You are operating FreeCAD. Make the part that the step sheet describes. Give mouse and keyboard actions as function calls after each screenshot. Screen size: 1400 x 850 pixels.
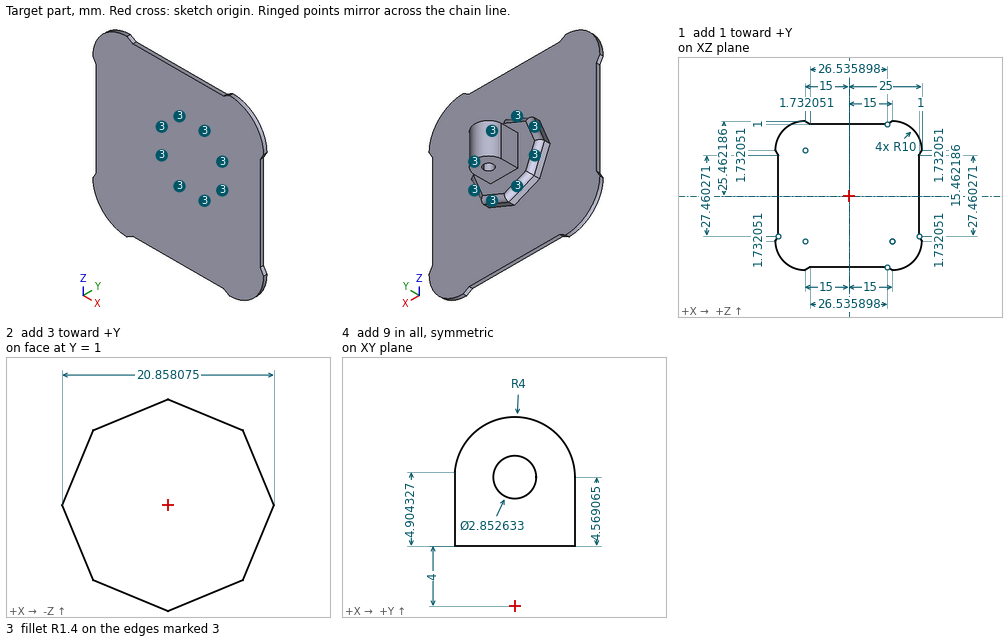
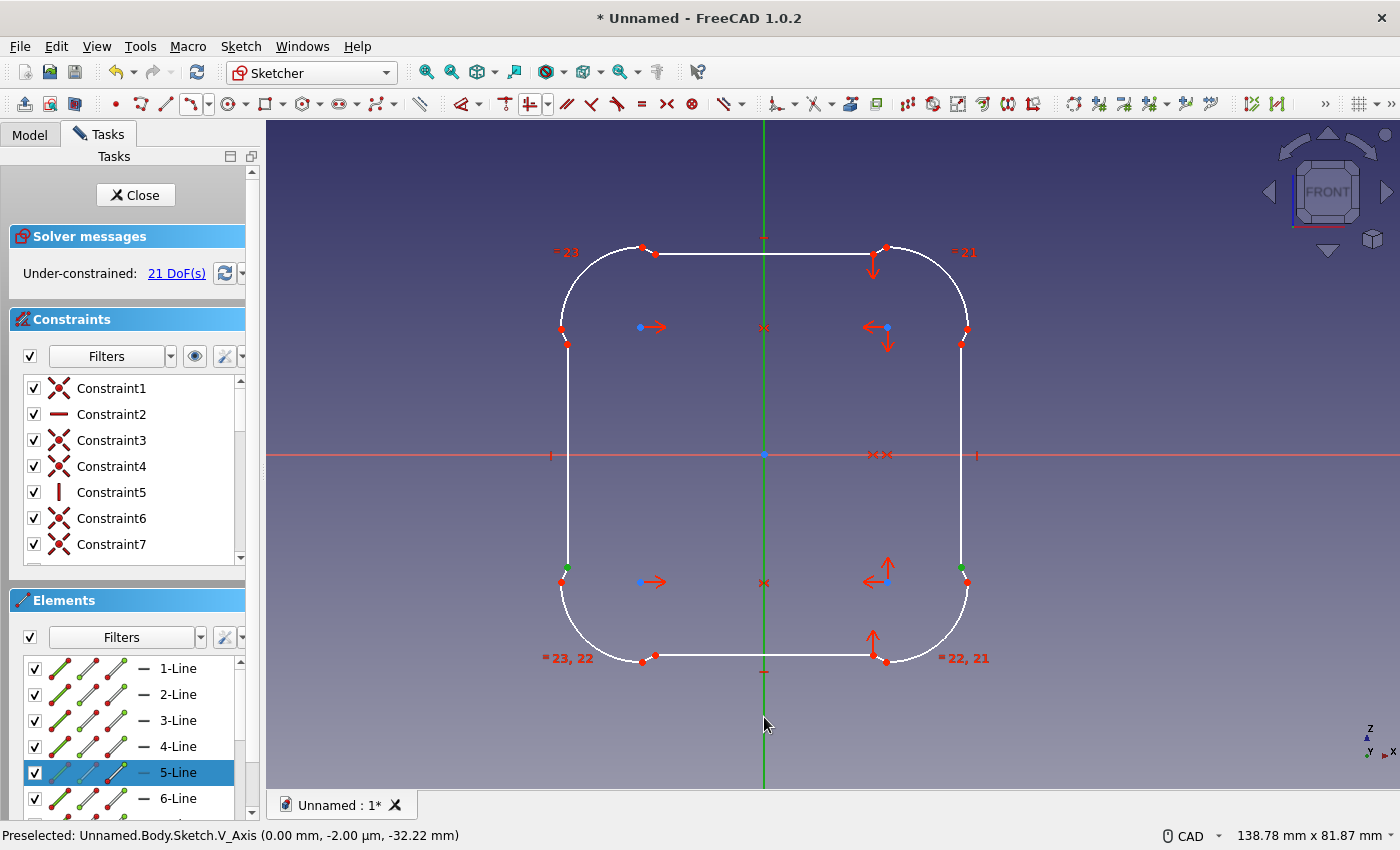
click(667, 104)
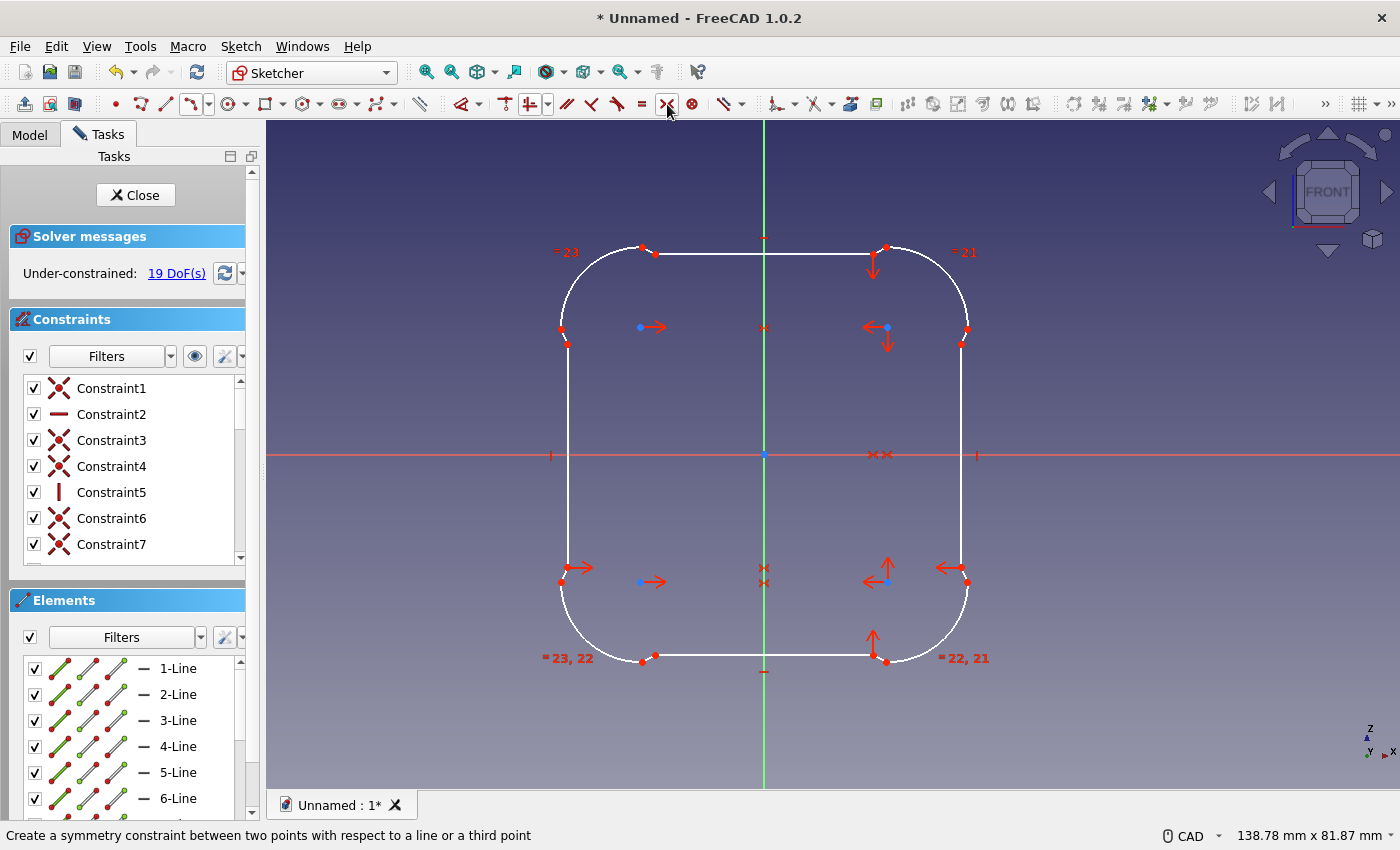
click(460, 104)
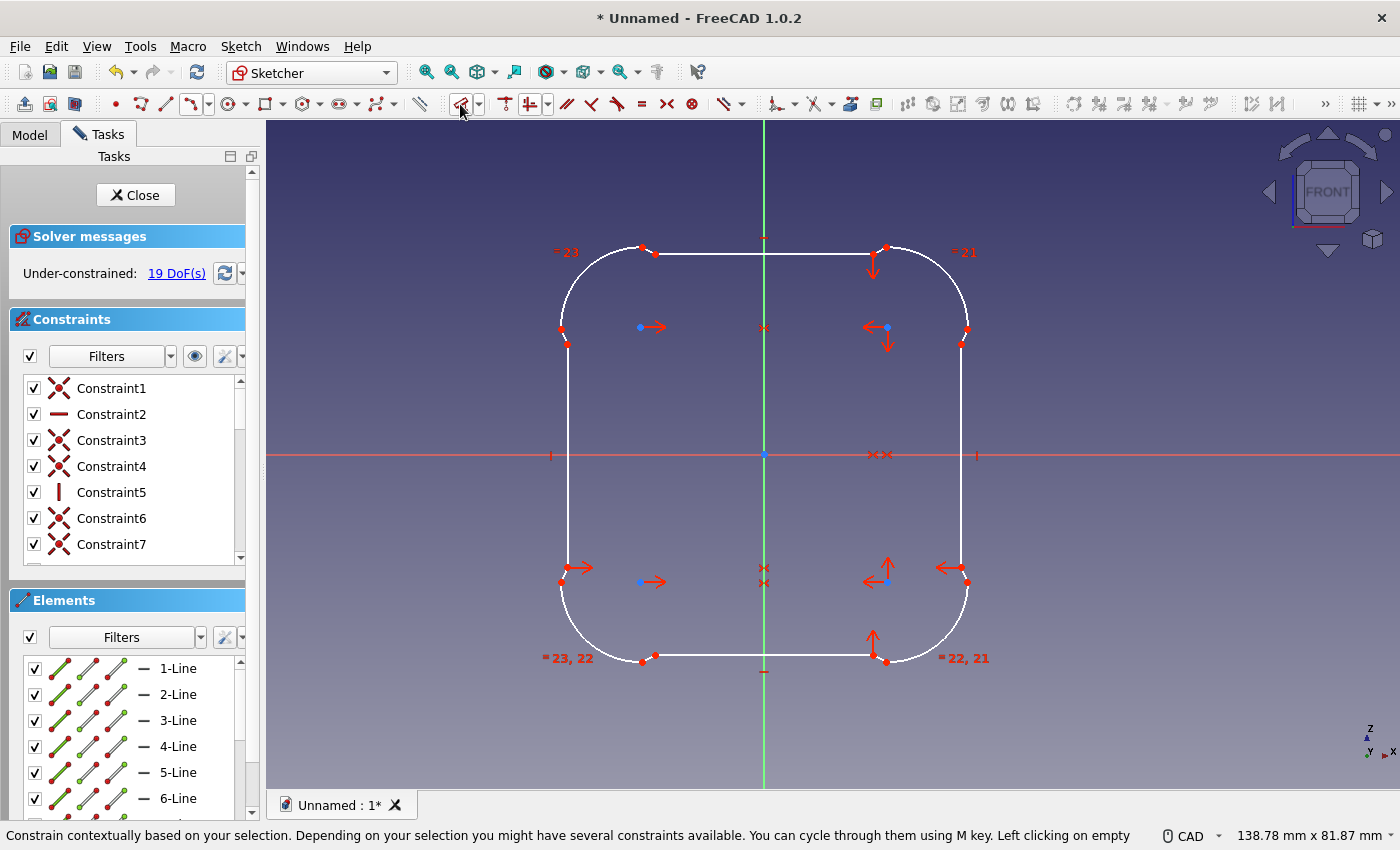
click(960, 292)
click(989, 278)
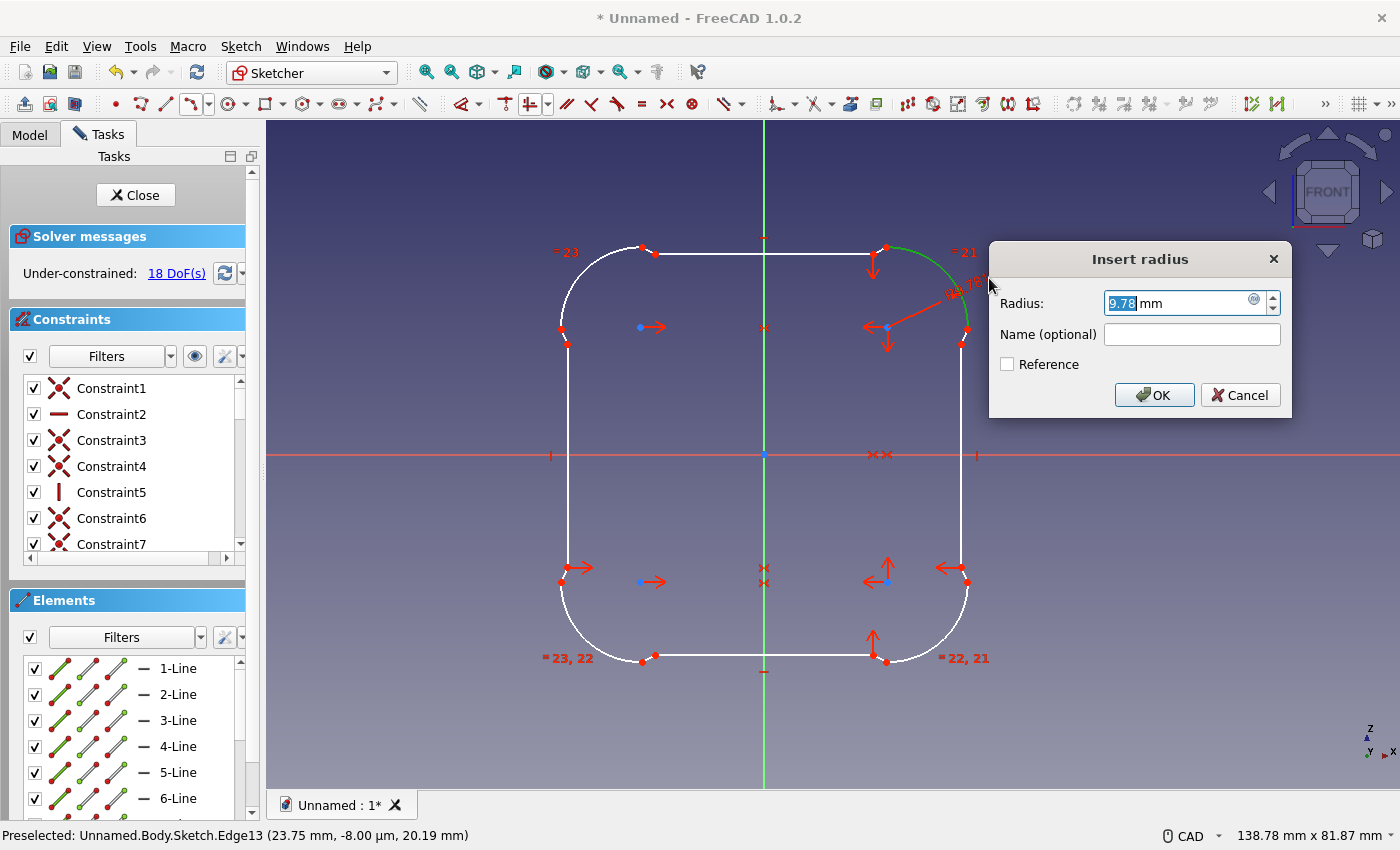
text(10)
key(Return)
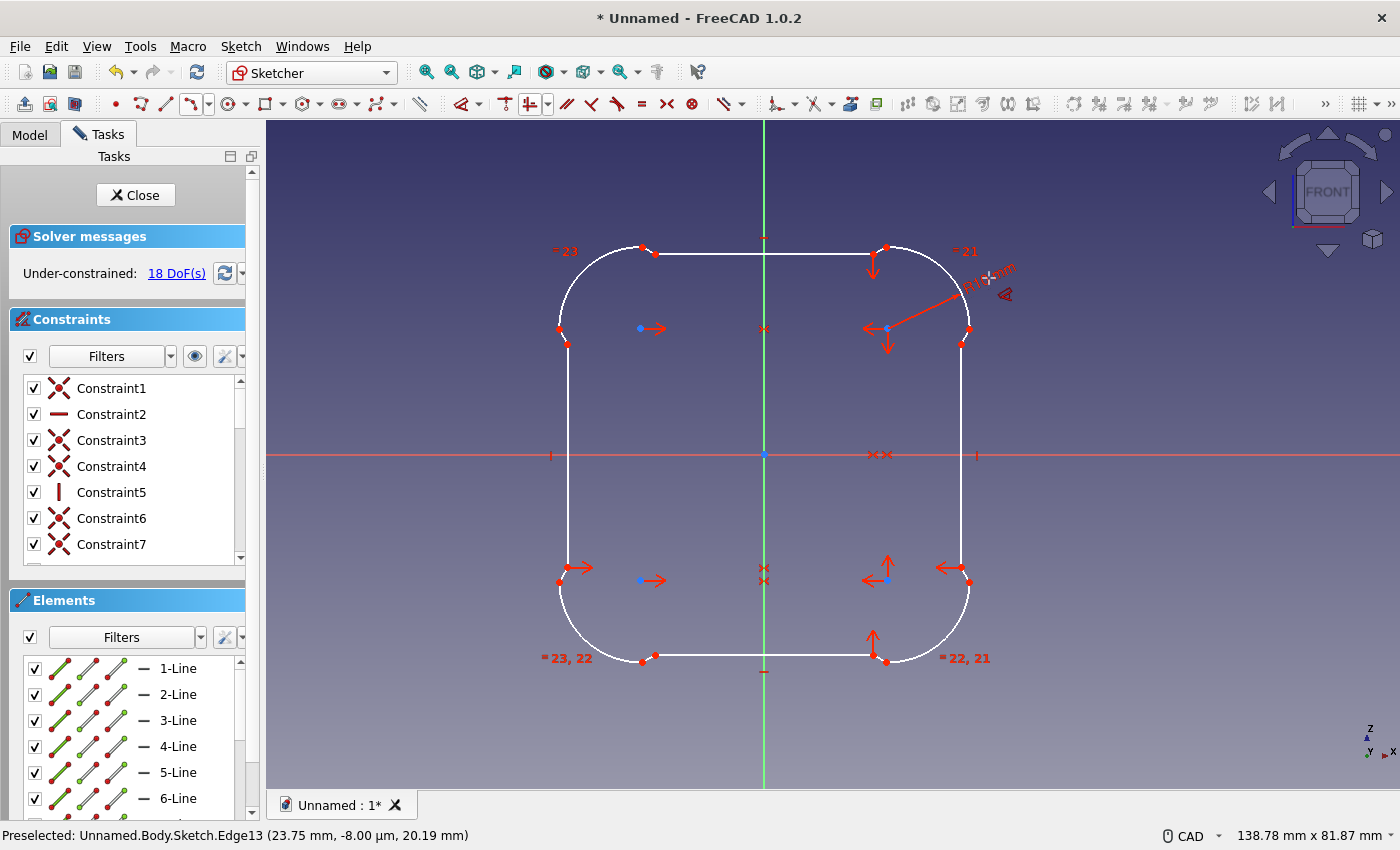
scroll(649, 251, up, 8)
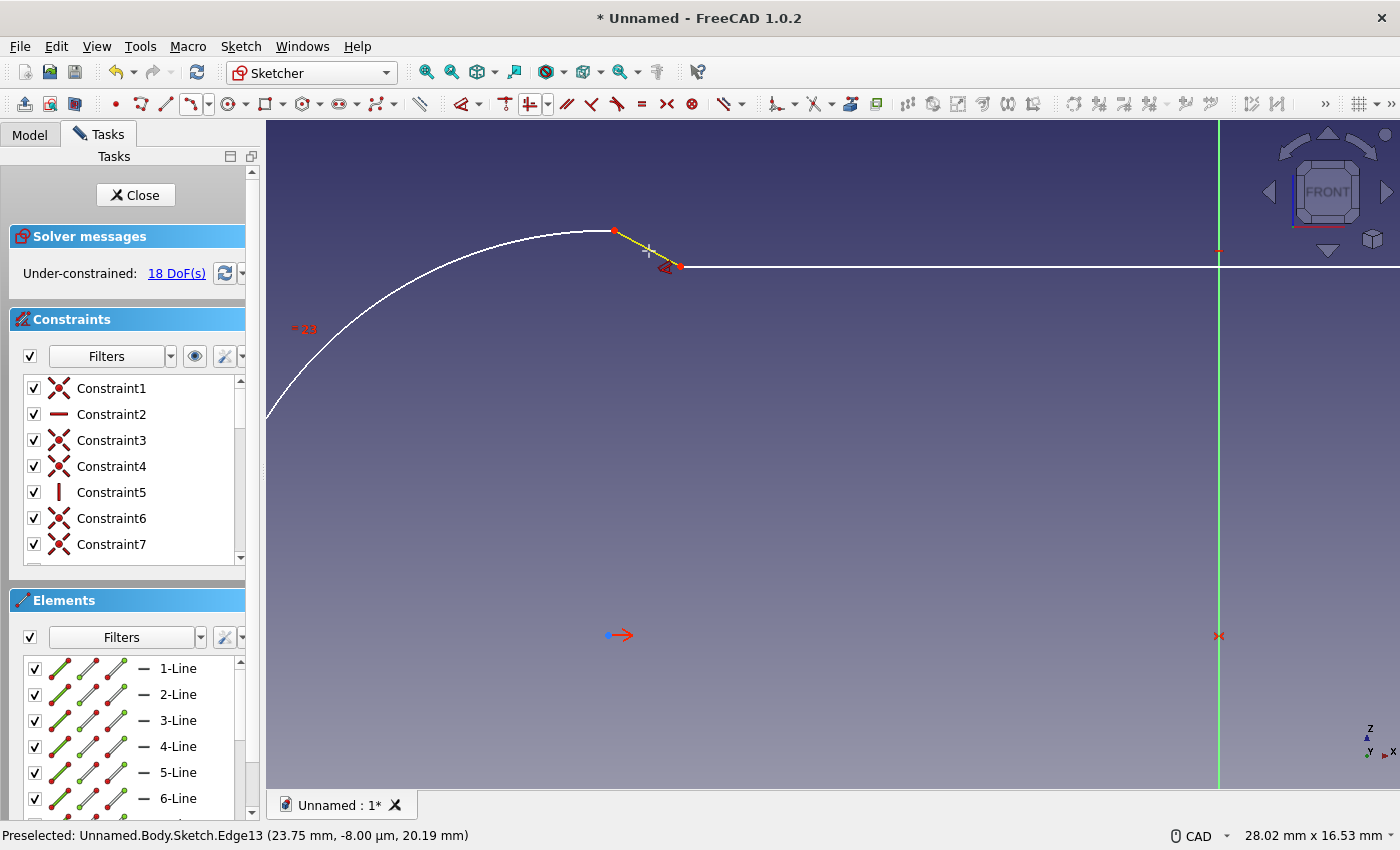
click(648, 249)
click(580, 249)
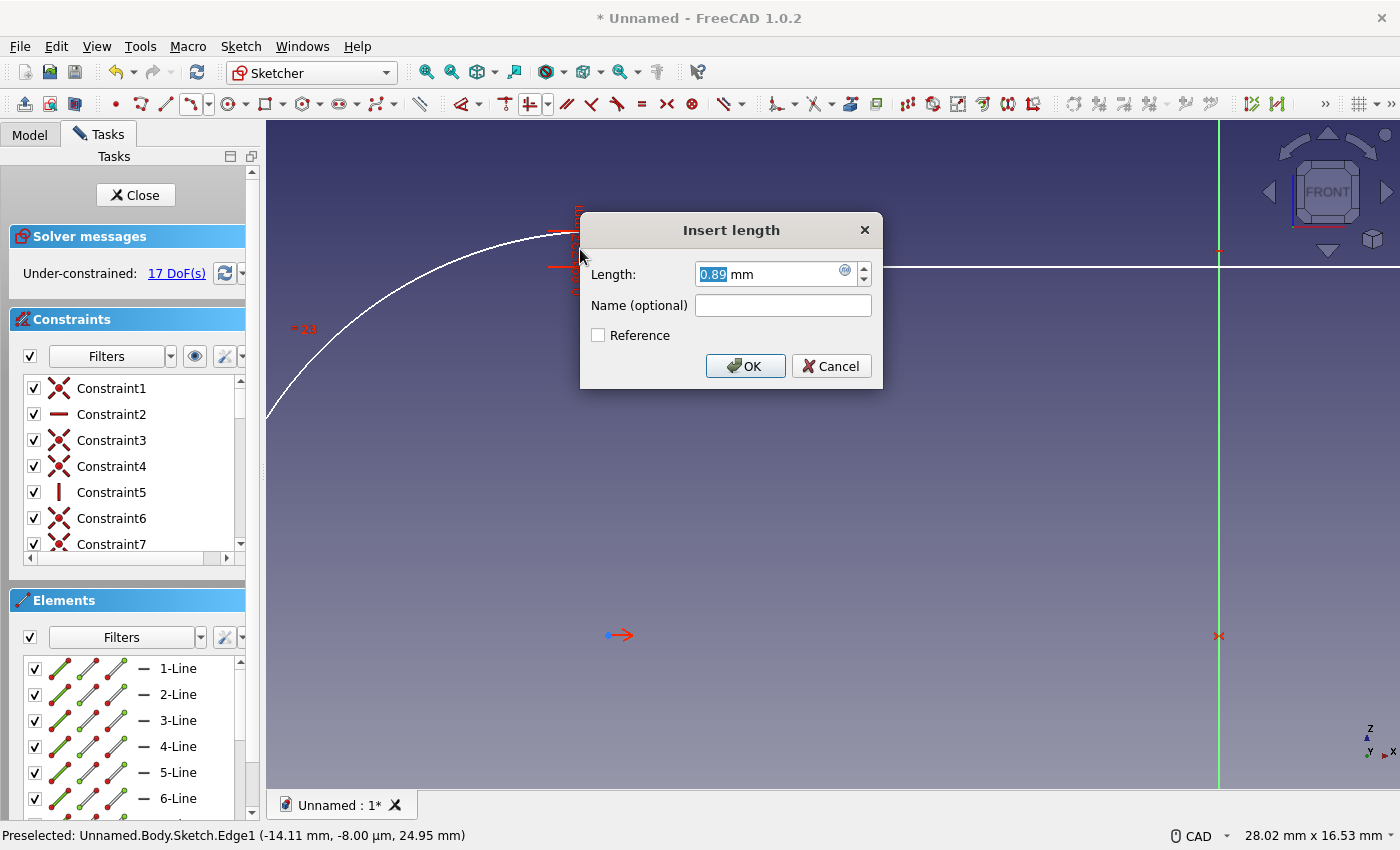
text(1)
key(Return)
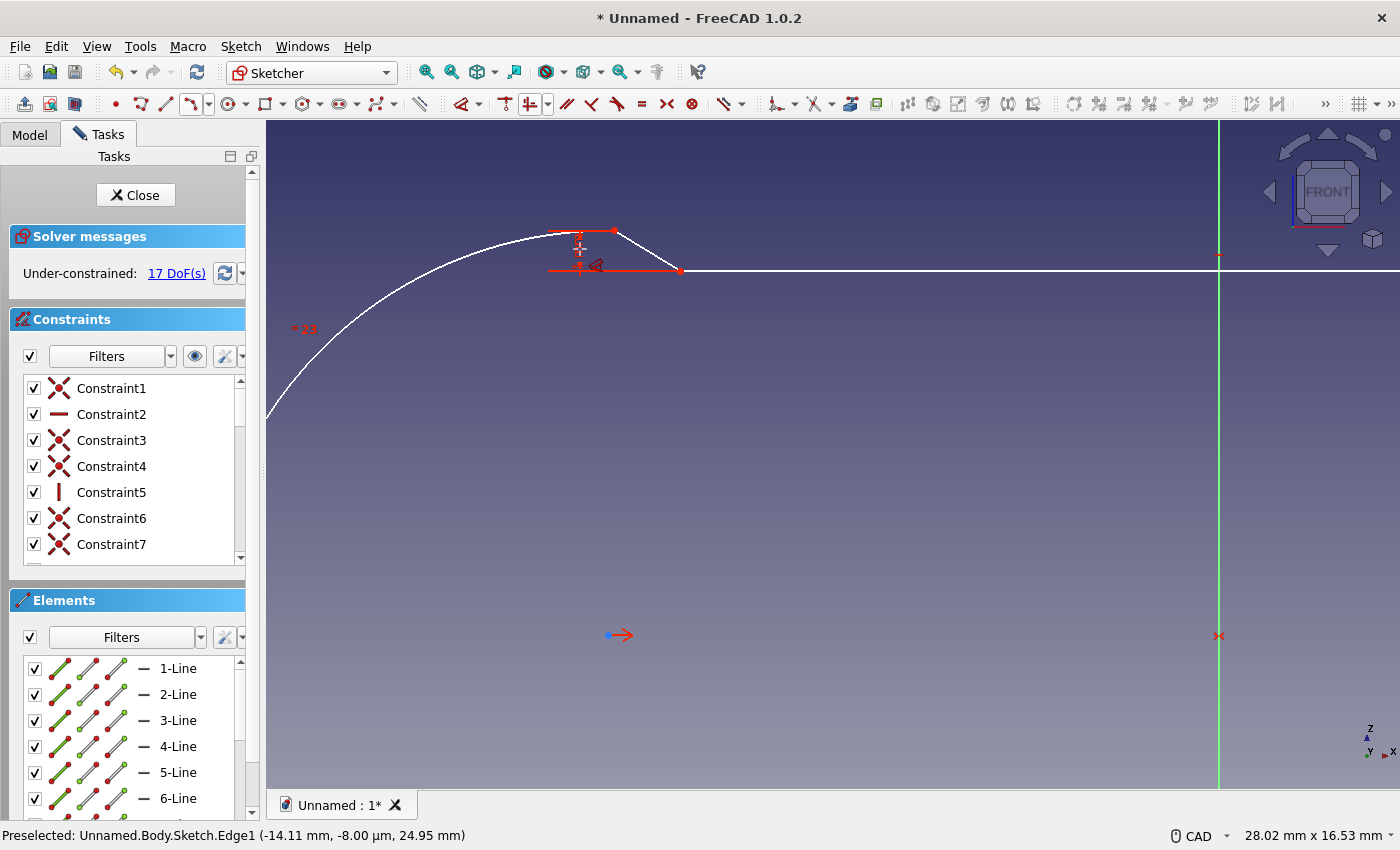
scroll(649, 251, down, 8)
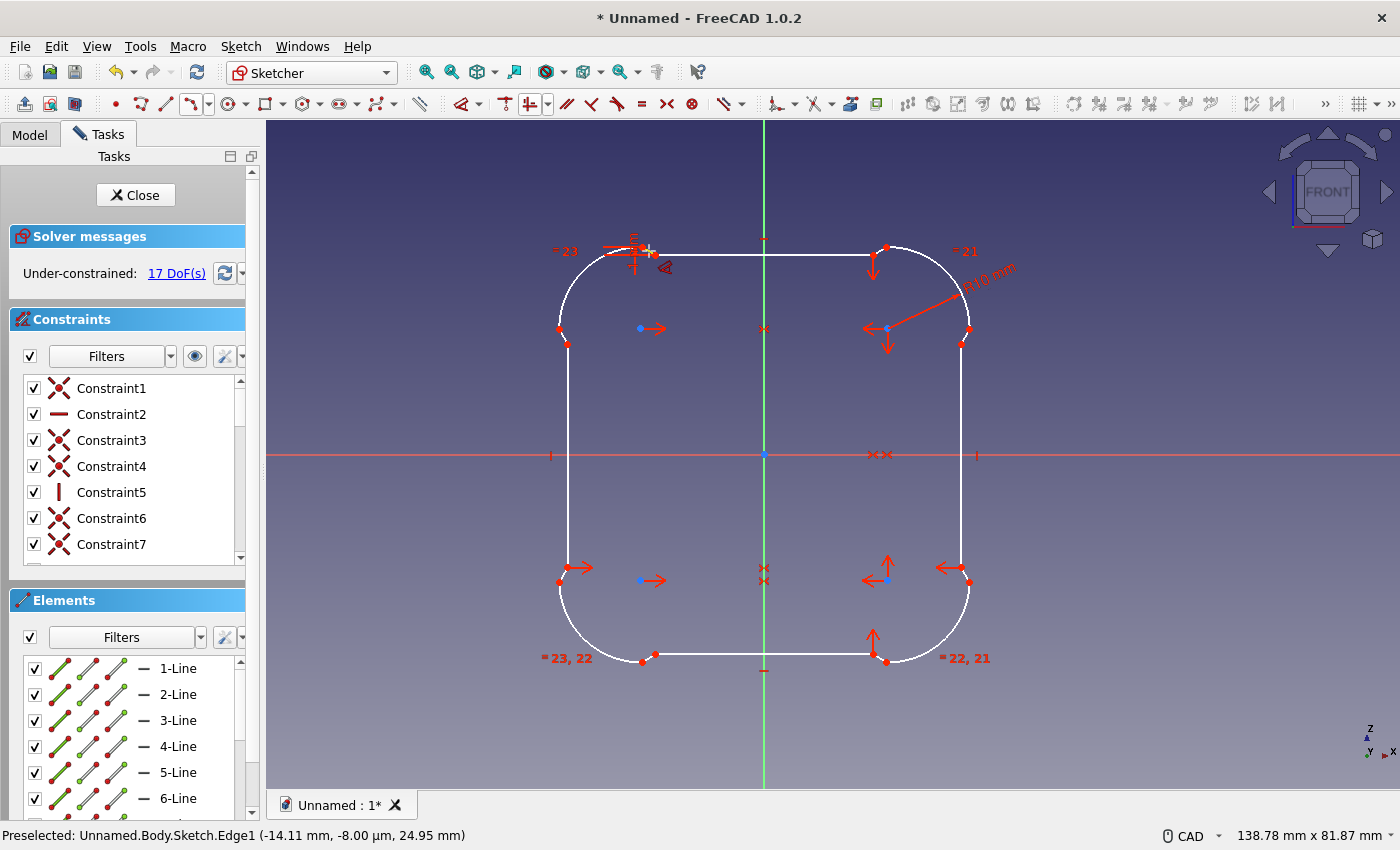
scroll(967, 334, up, 8)